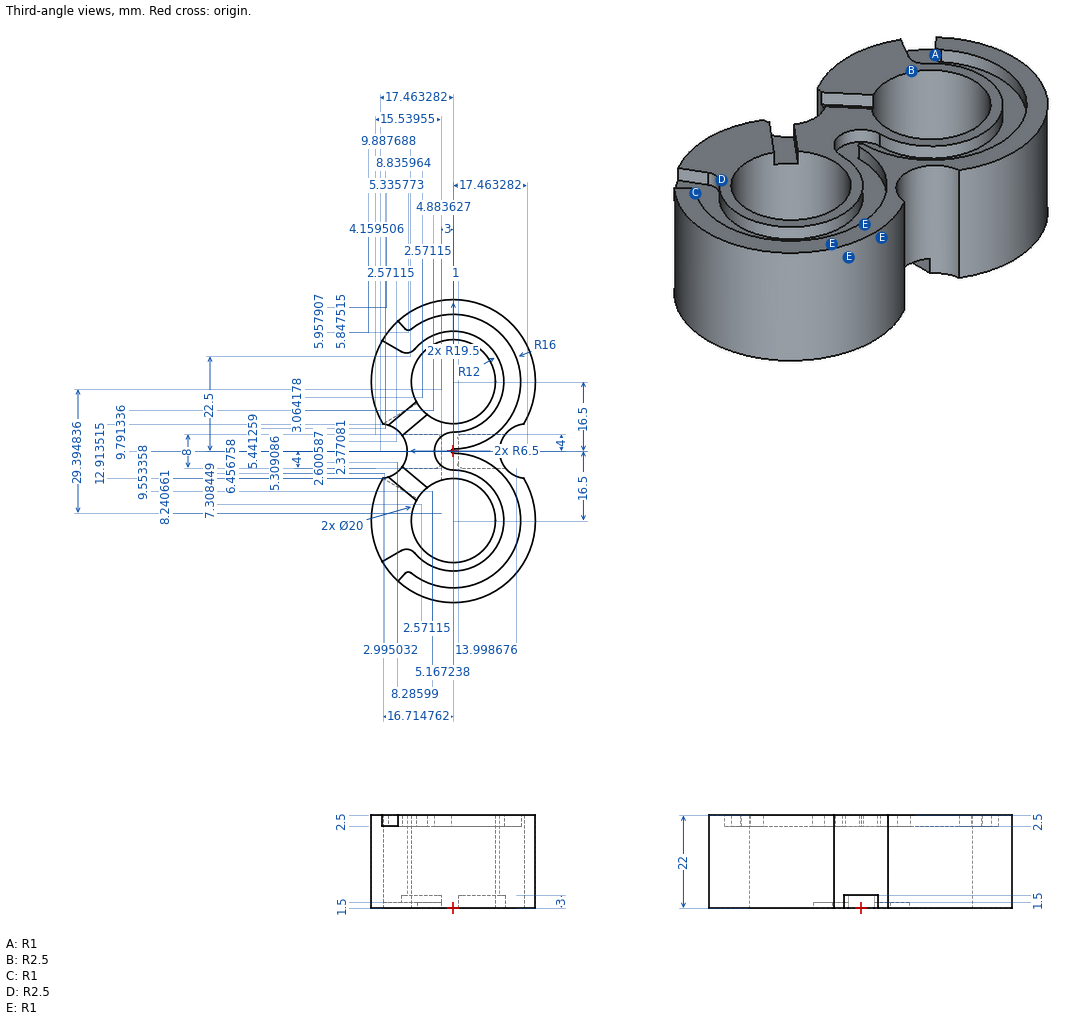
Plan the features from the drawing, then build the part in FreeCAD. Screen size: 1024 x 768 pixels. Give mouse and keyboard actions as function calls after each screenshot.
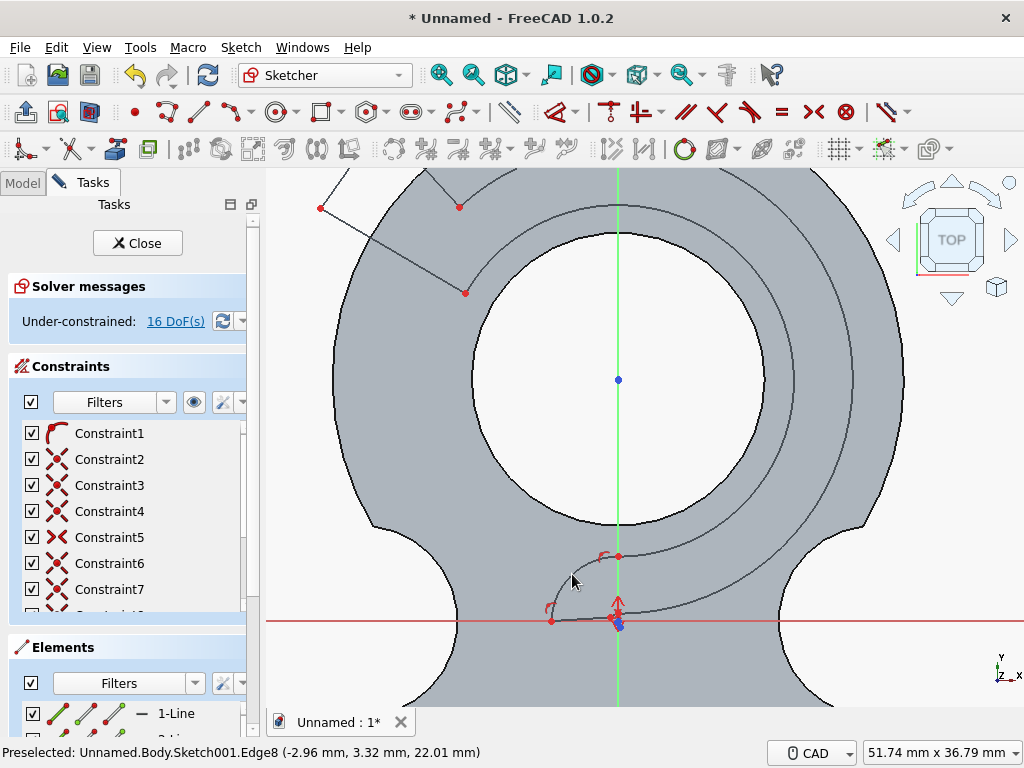
scroll(614, 615, up, 7)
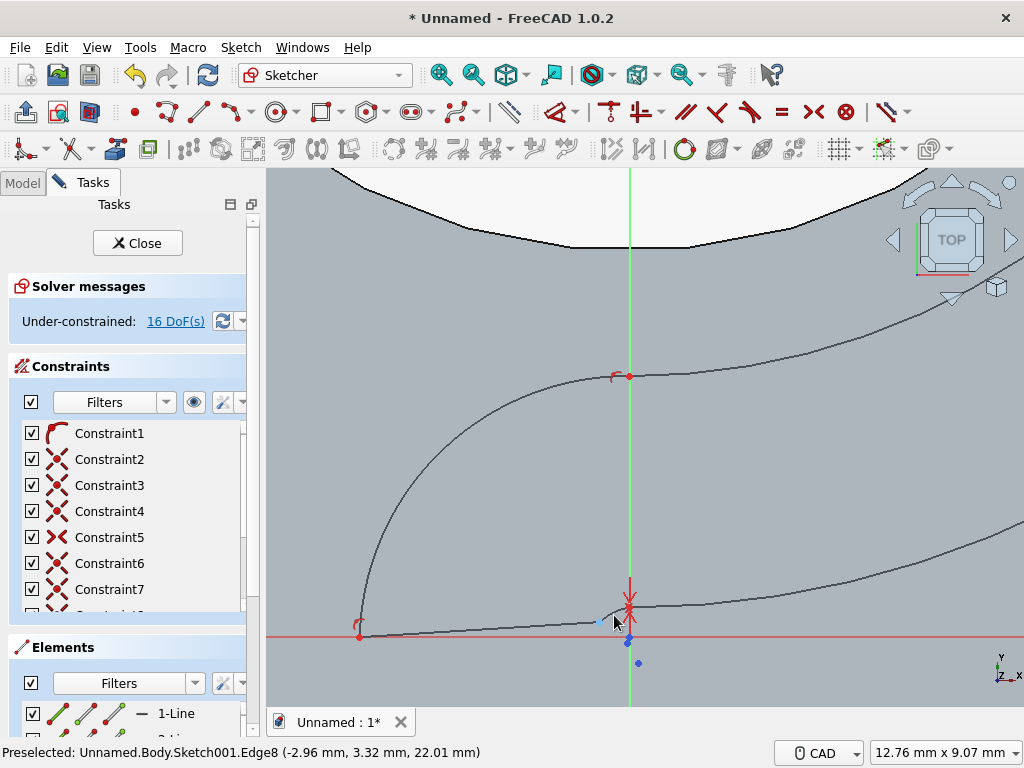
click(614, 613)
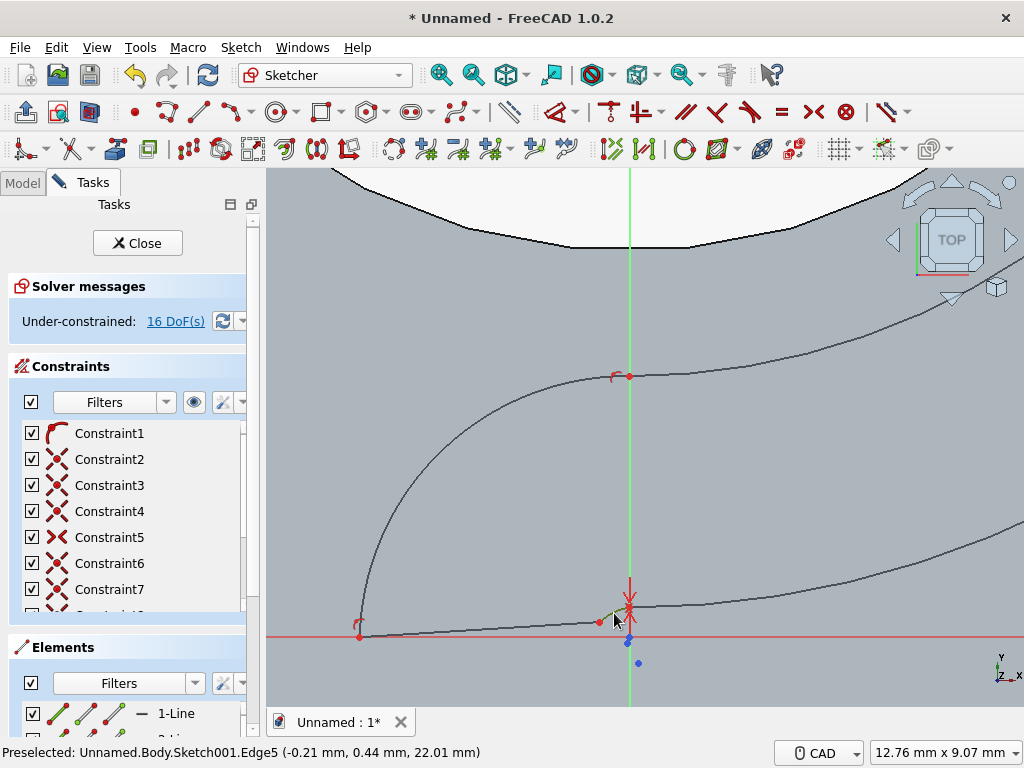
scroll(598, 599, down, 9)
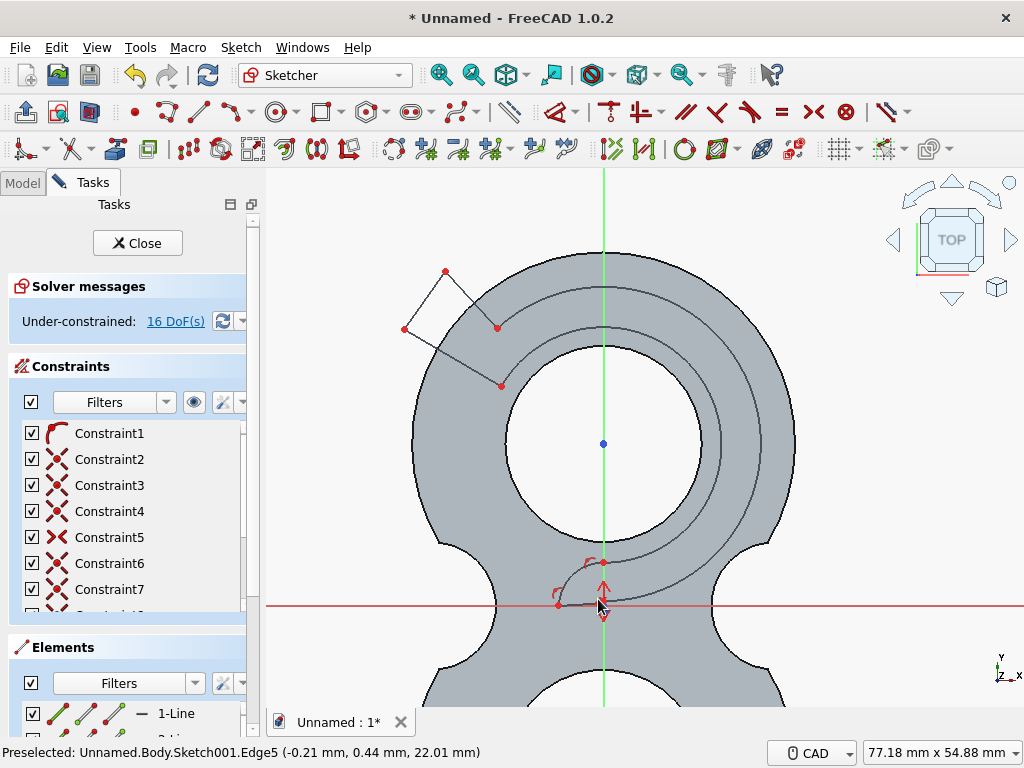
click(748, 506)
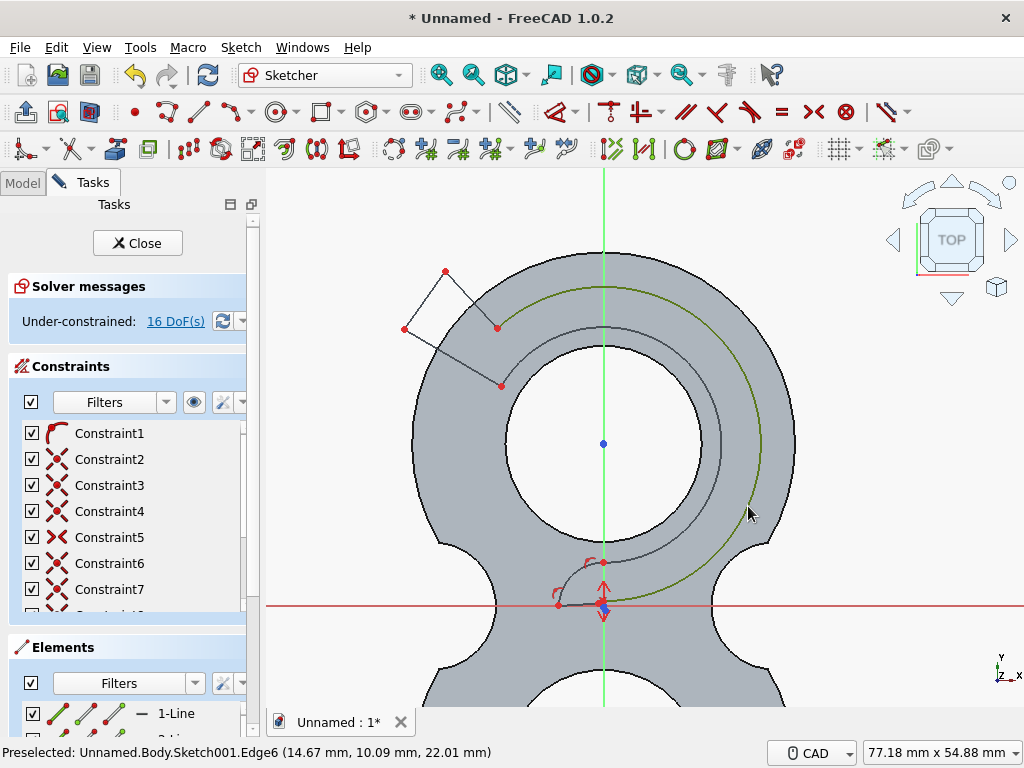
click(750, 112)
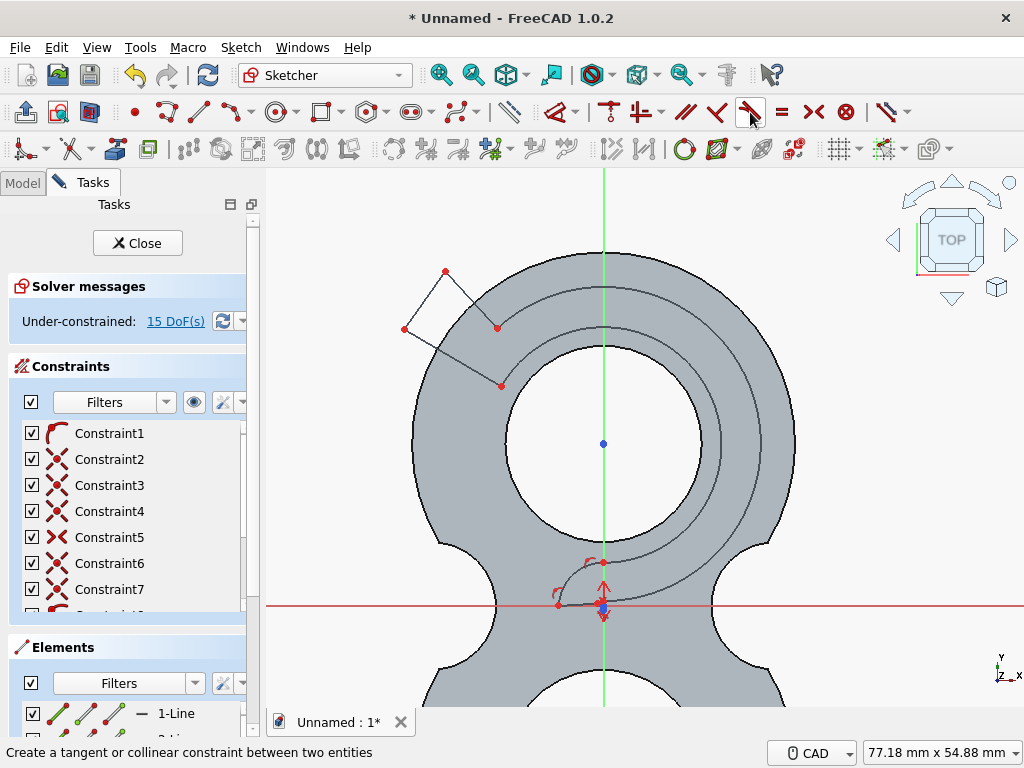
click(716, 481)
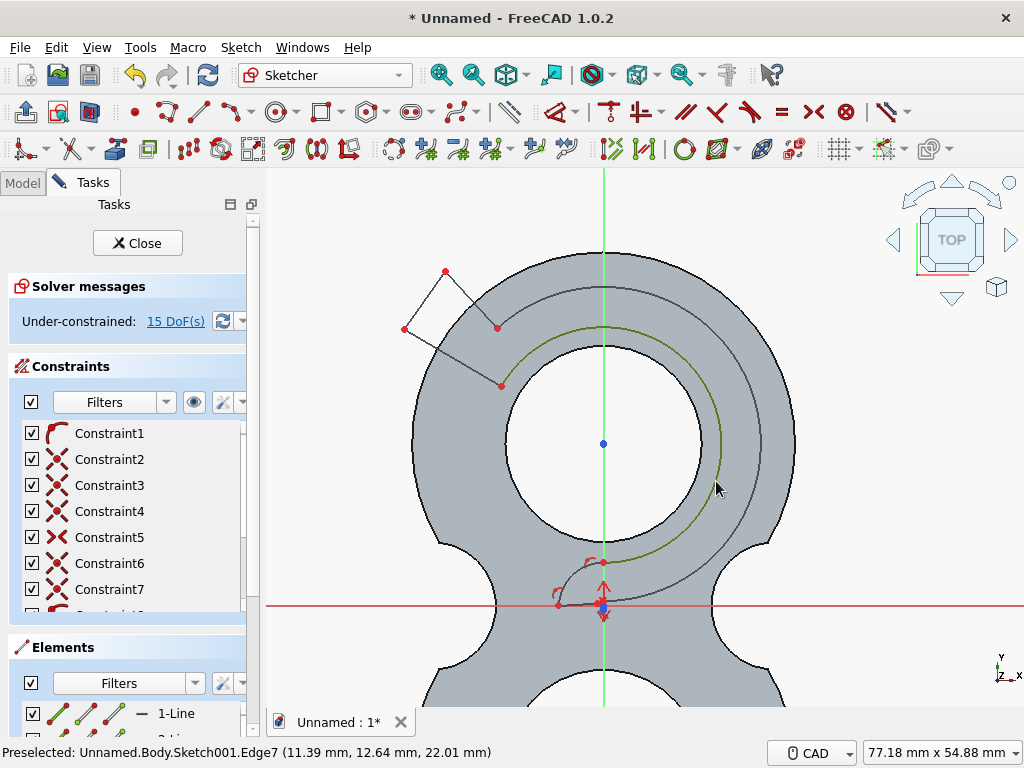
click(584, 567)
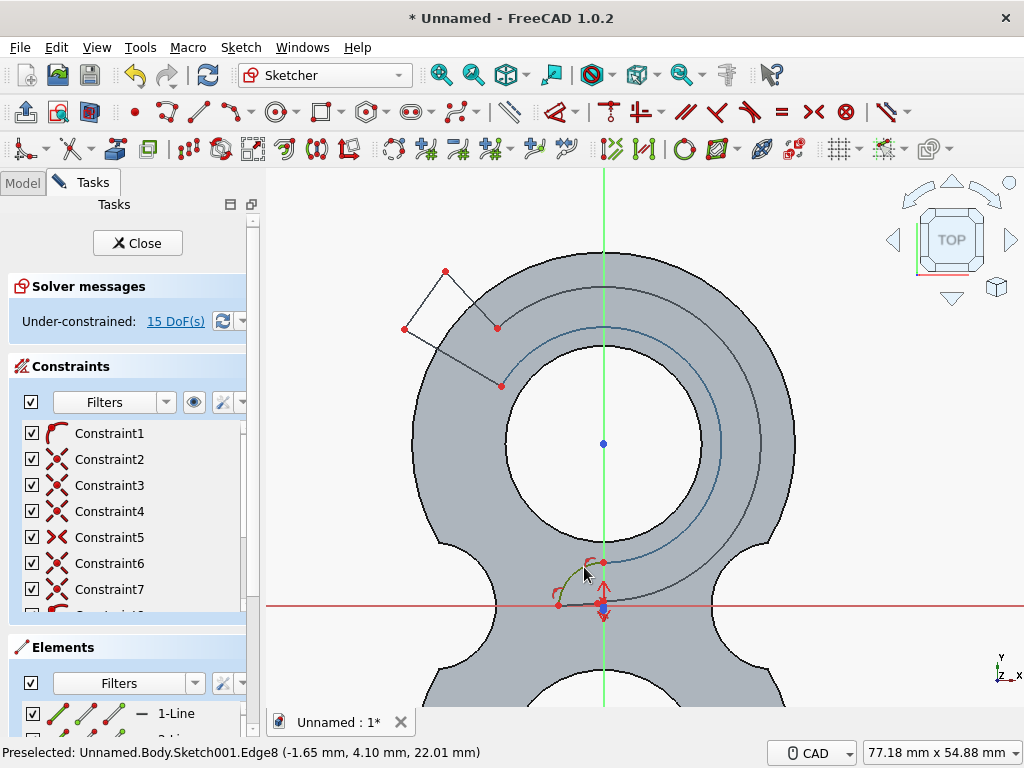
key(t)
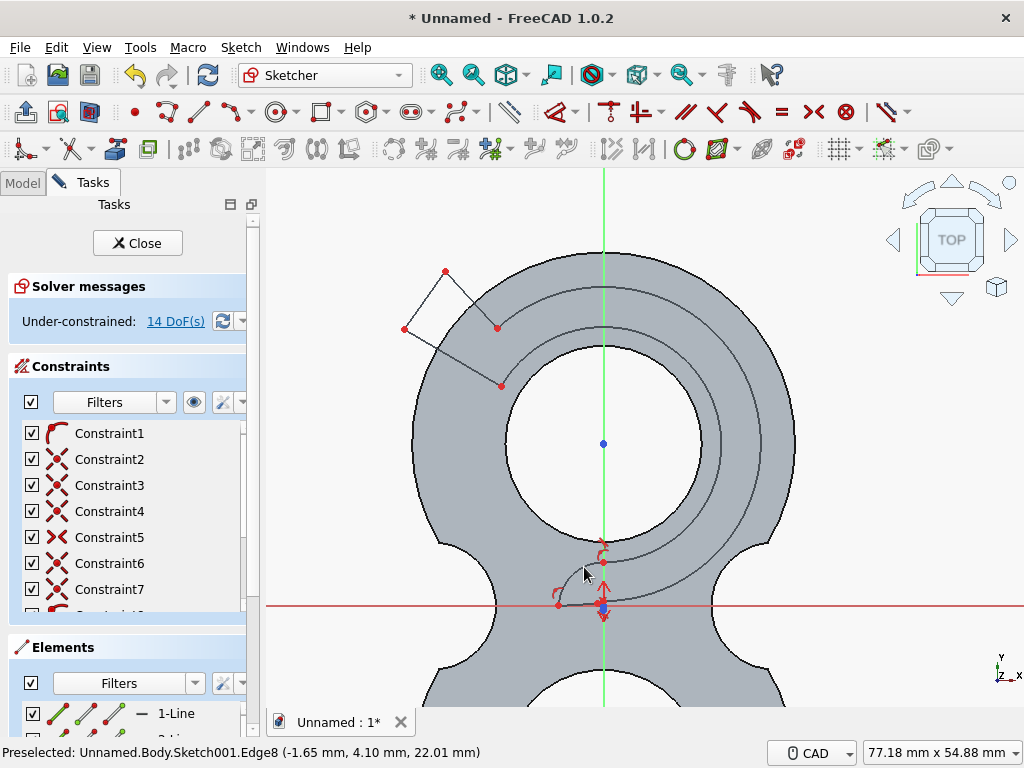
click(570, 605)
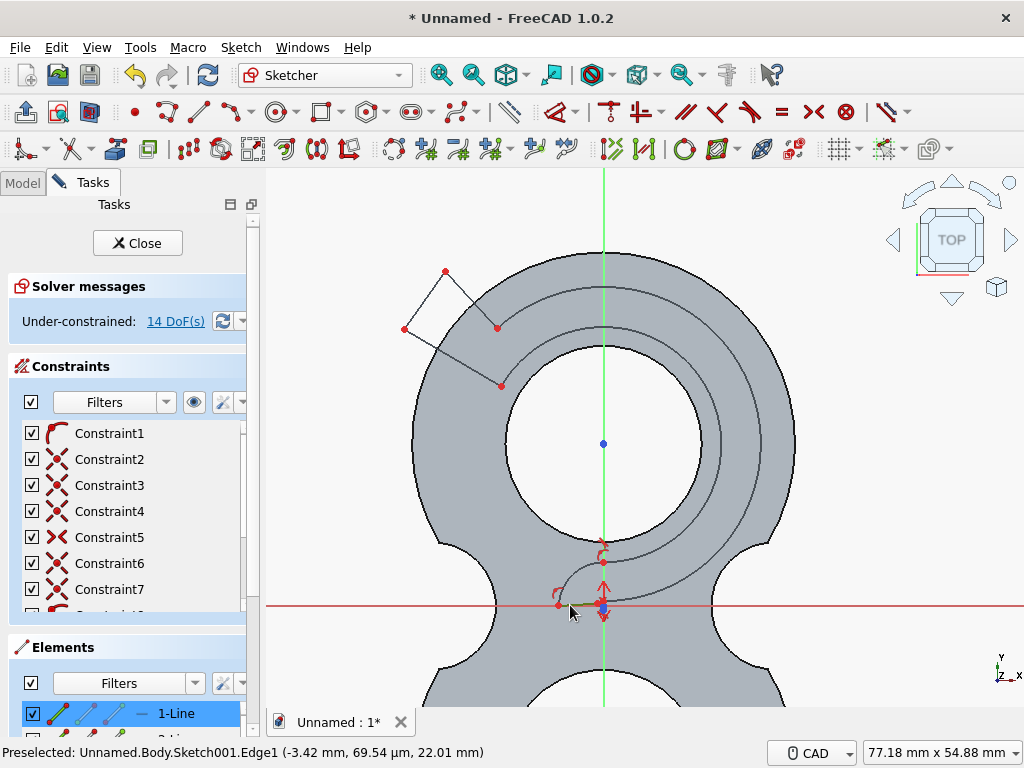
key(h)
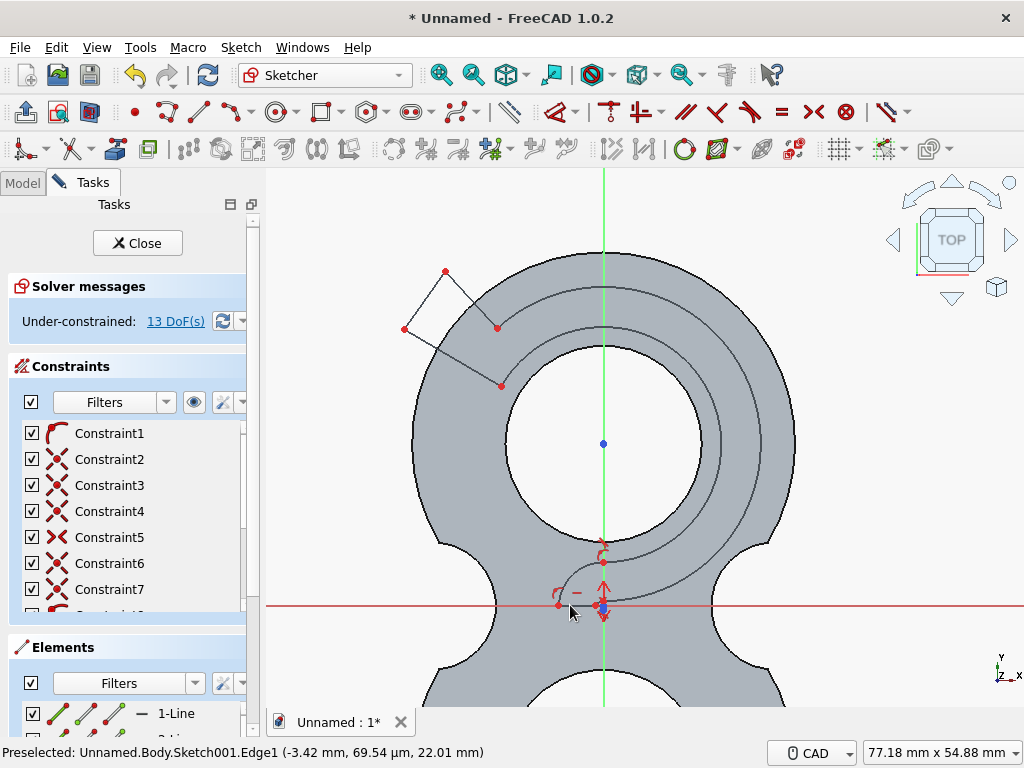
click(748, 506)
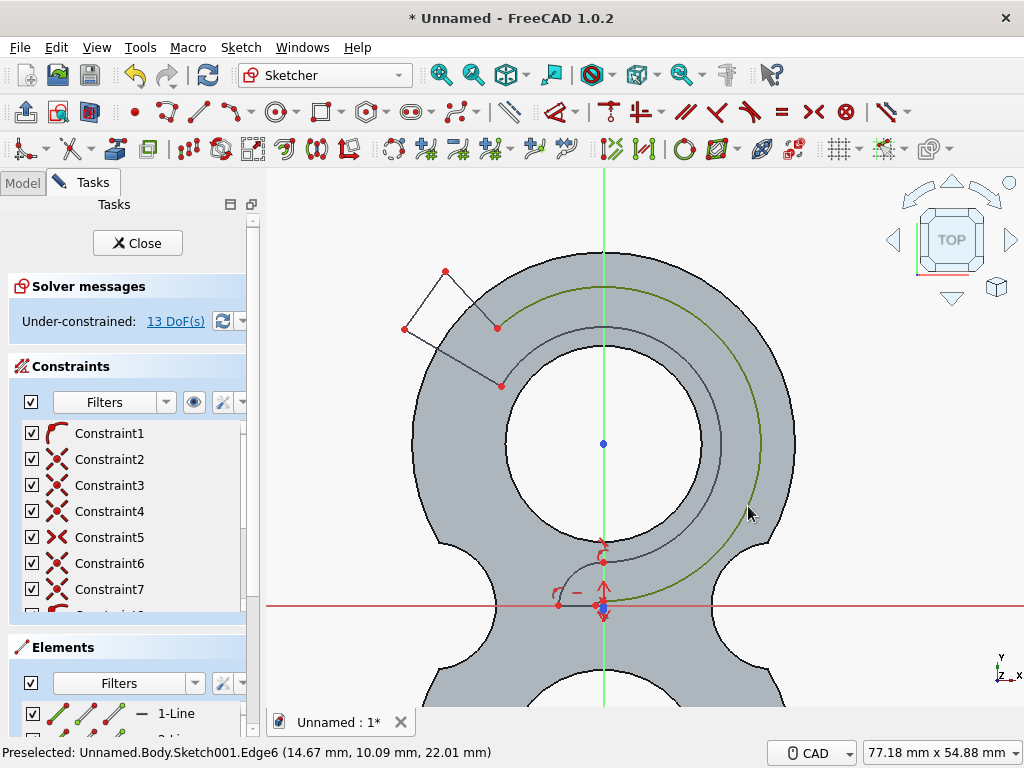
click(716, 481)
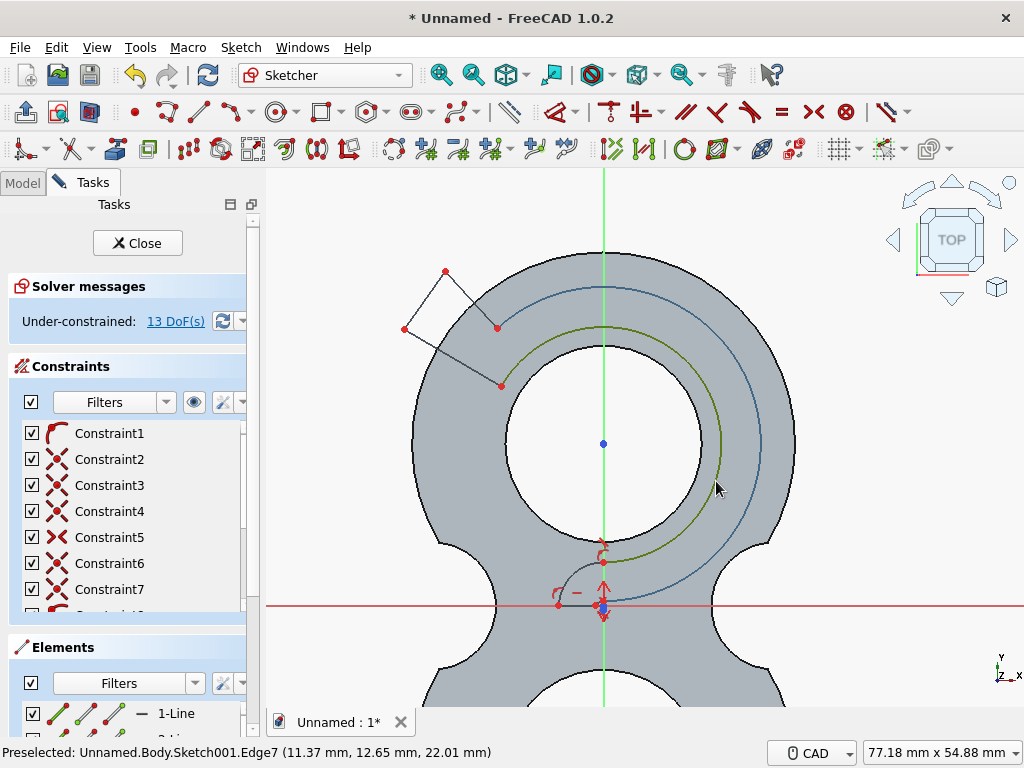
click(610, 112)